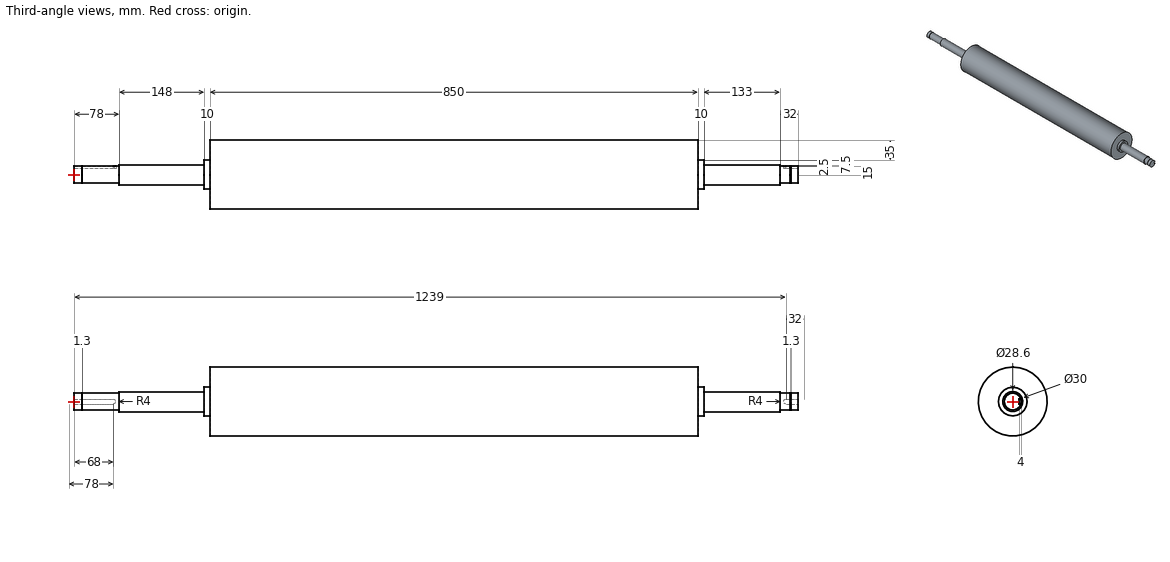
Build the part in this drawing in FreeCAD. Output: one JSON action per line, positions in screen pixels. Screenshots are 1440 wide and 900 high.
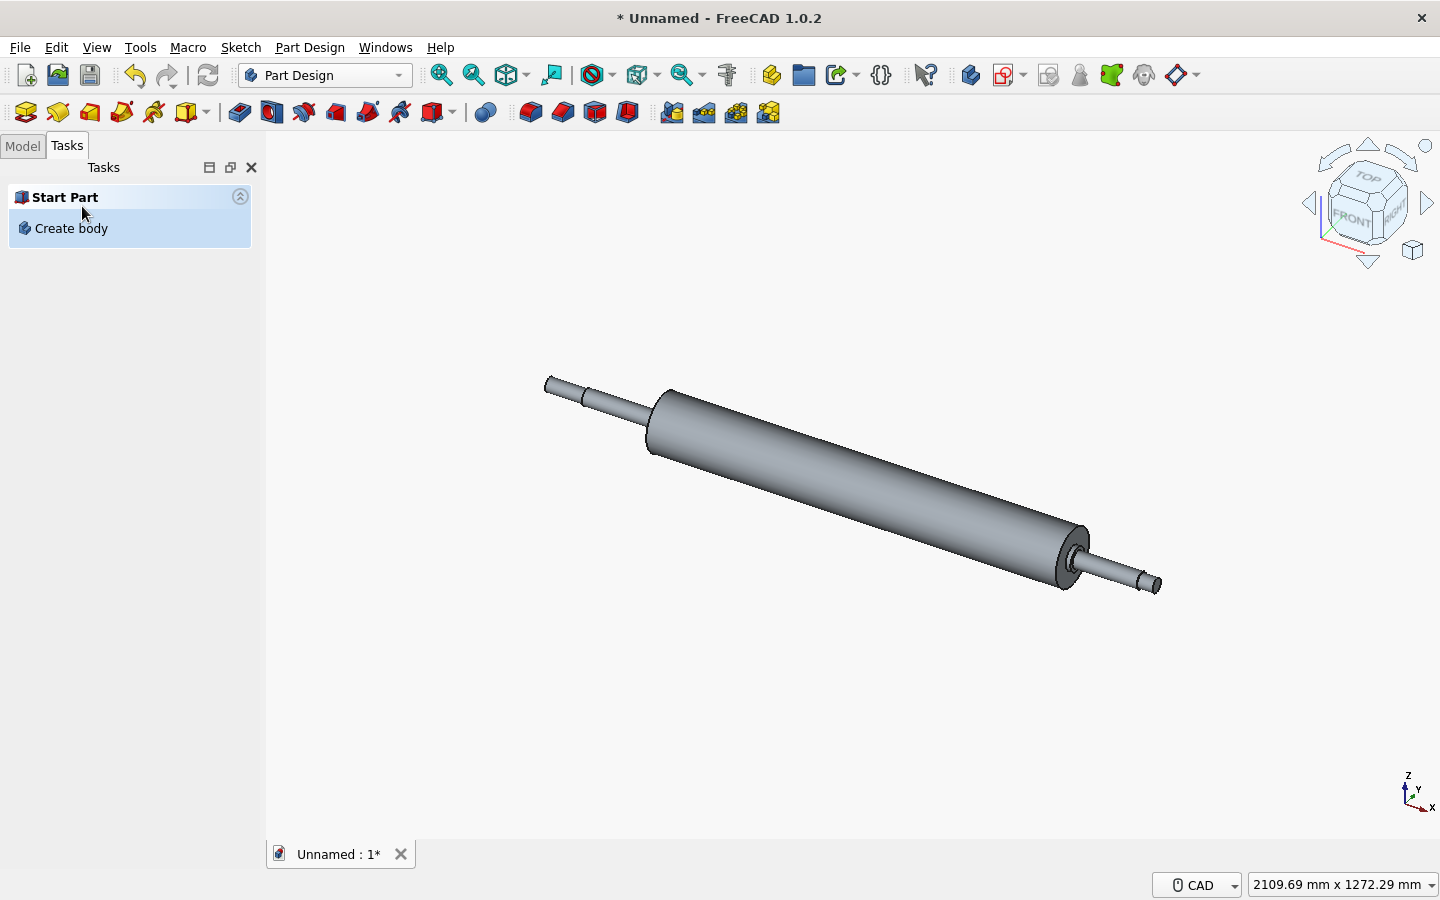
{"action": "left_click", "coordinate": [23, 145]}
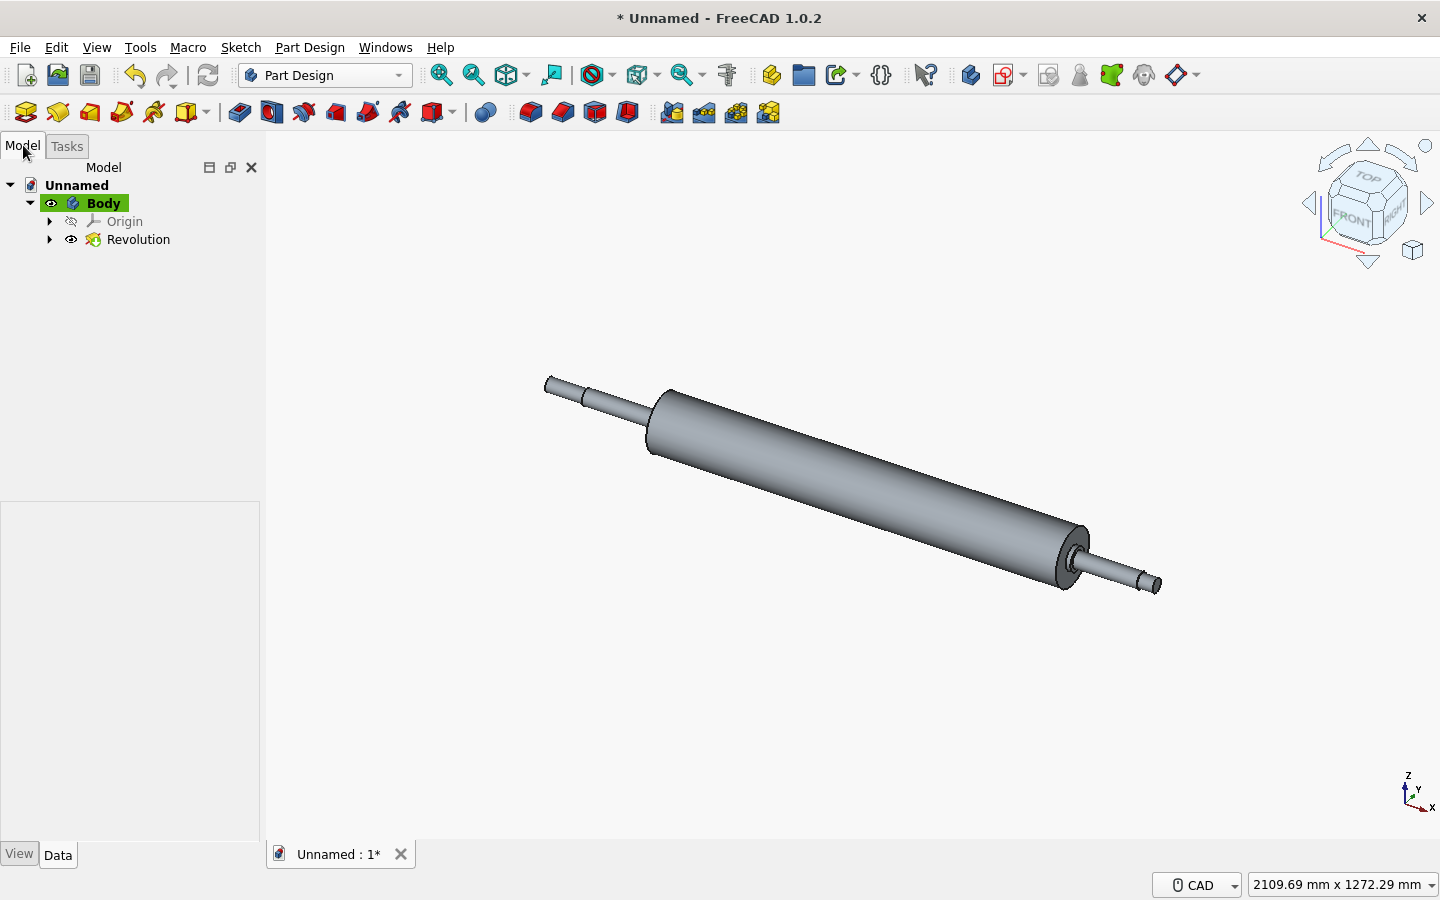
{"action": "left_click", "coordinate": [50, 221]}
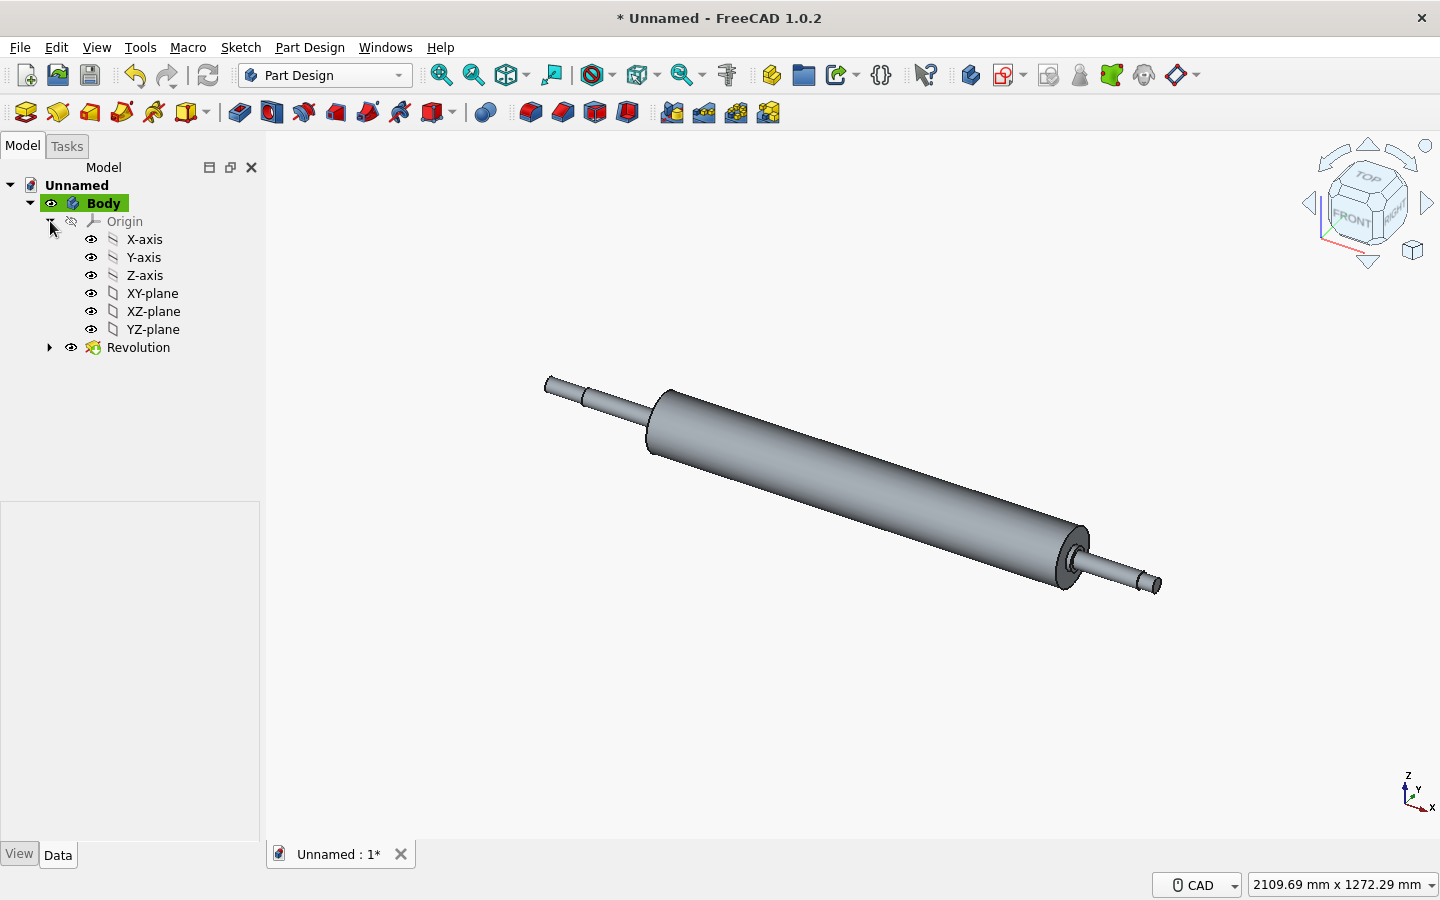
{"action": "left_click", "coordinate": [136, 311]}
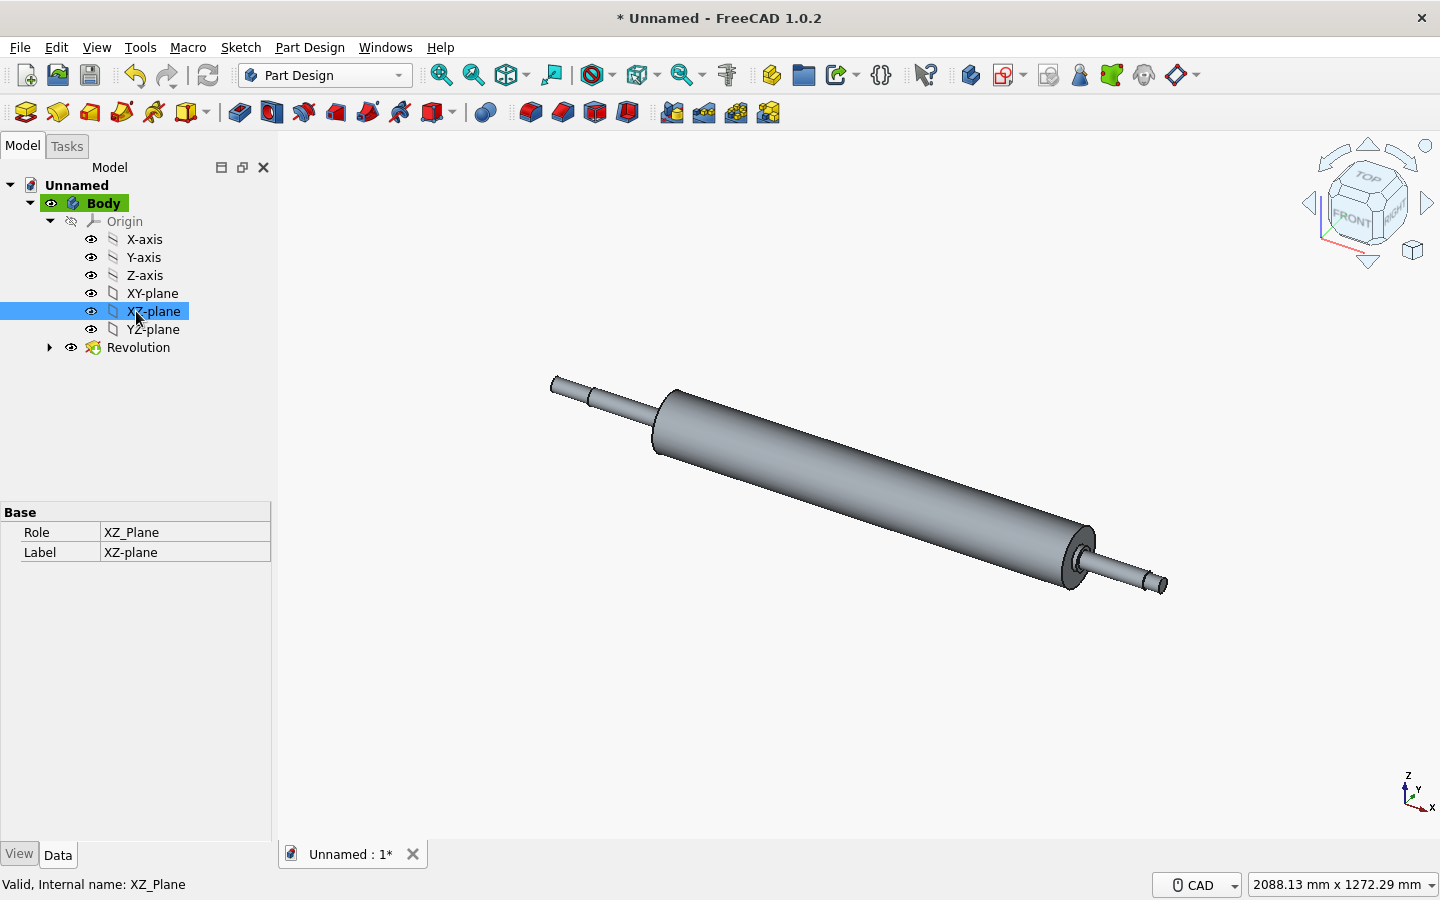
{"action": "left_click", "coordinate": [1176, 76]}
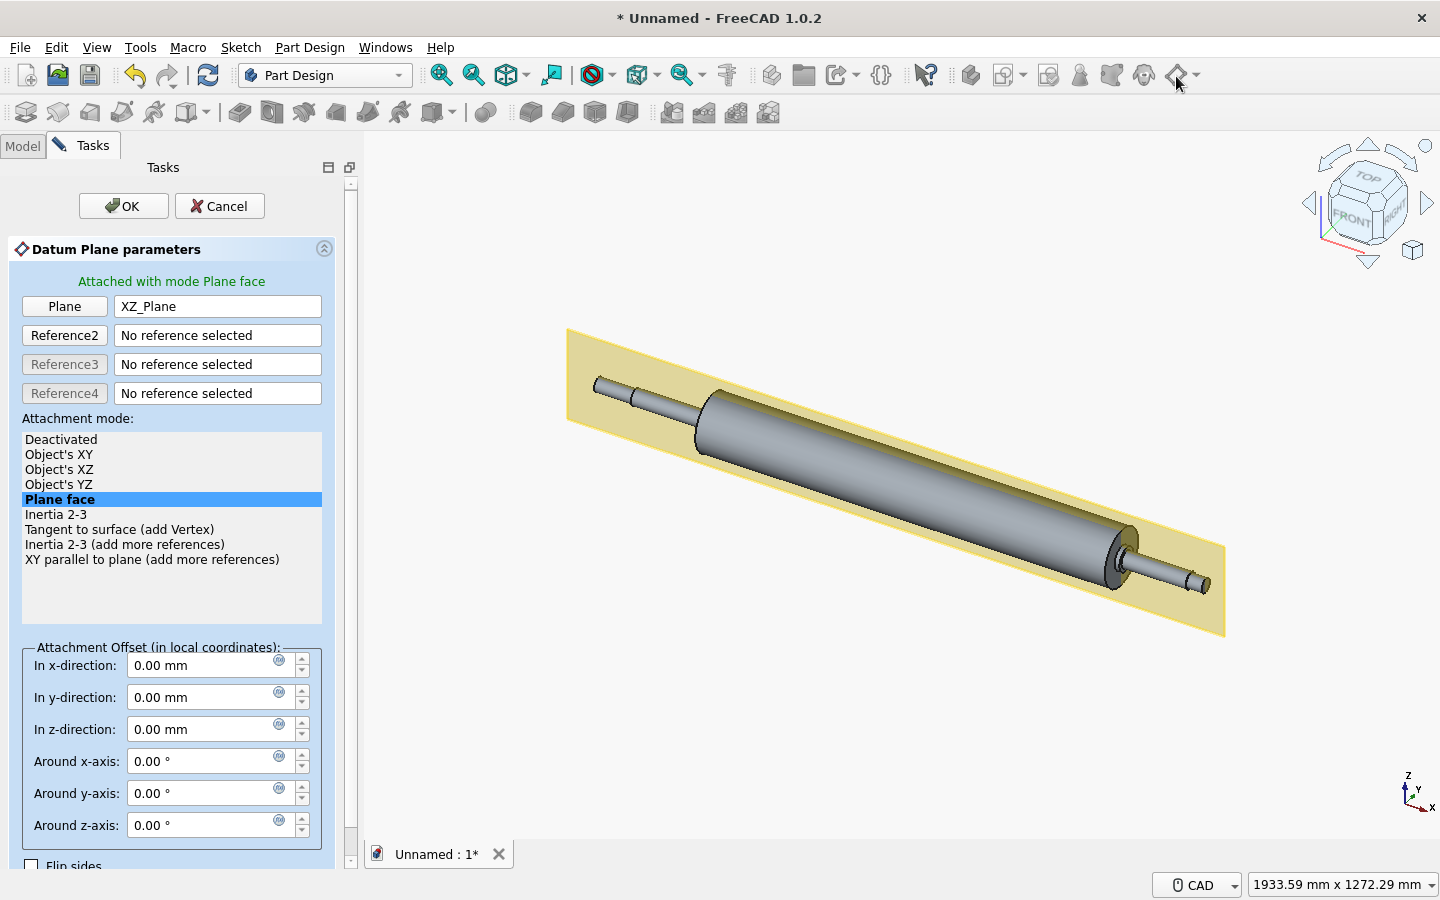
{"action": "triple_click", "coordinate": [210, 729]}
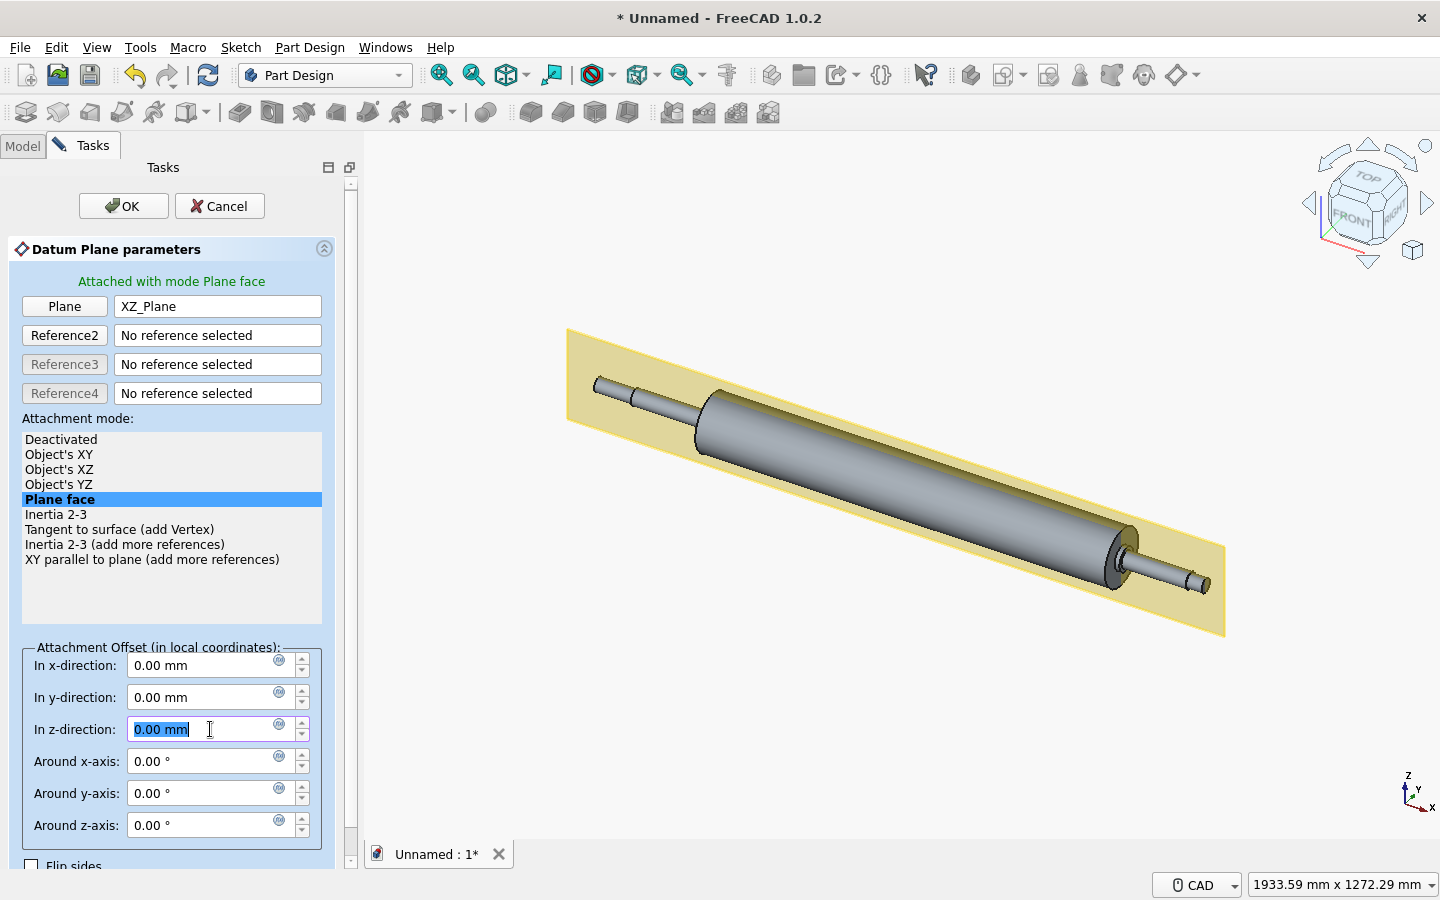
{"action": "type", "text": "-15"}
{"action": "key", "text": "Tab"}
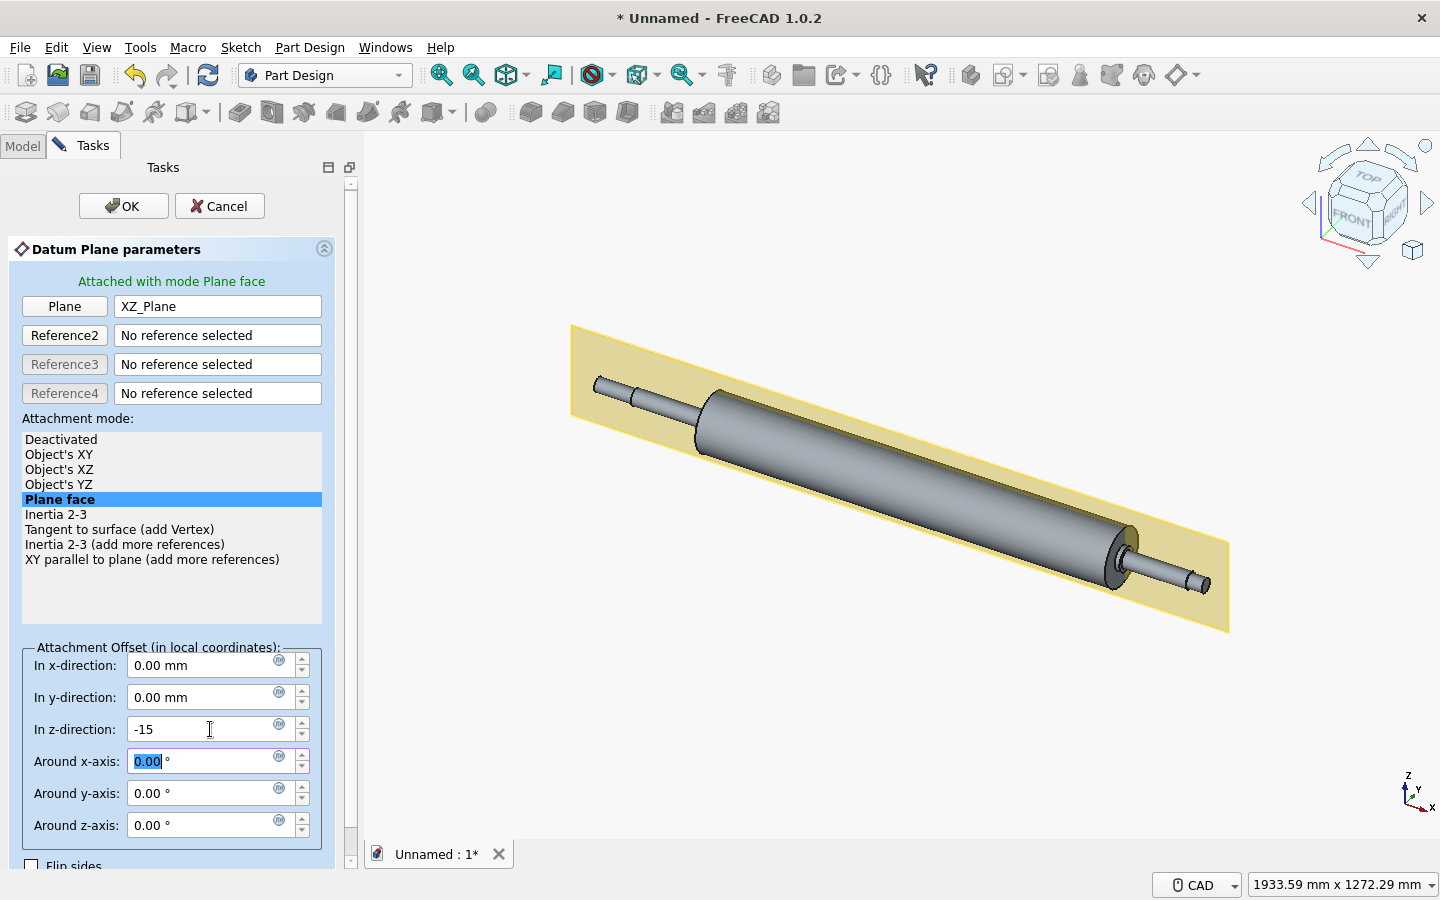
{"action": "left_click", "coordinate": [124, 206]}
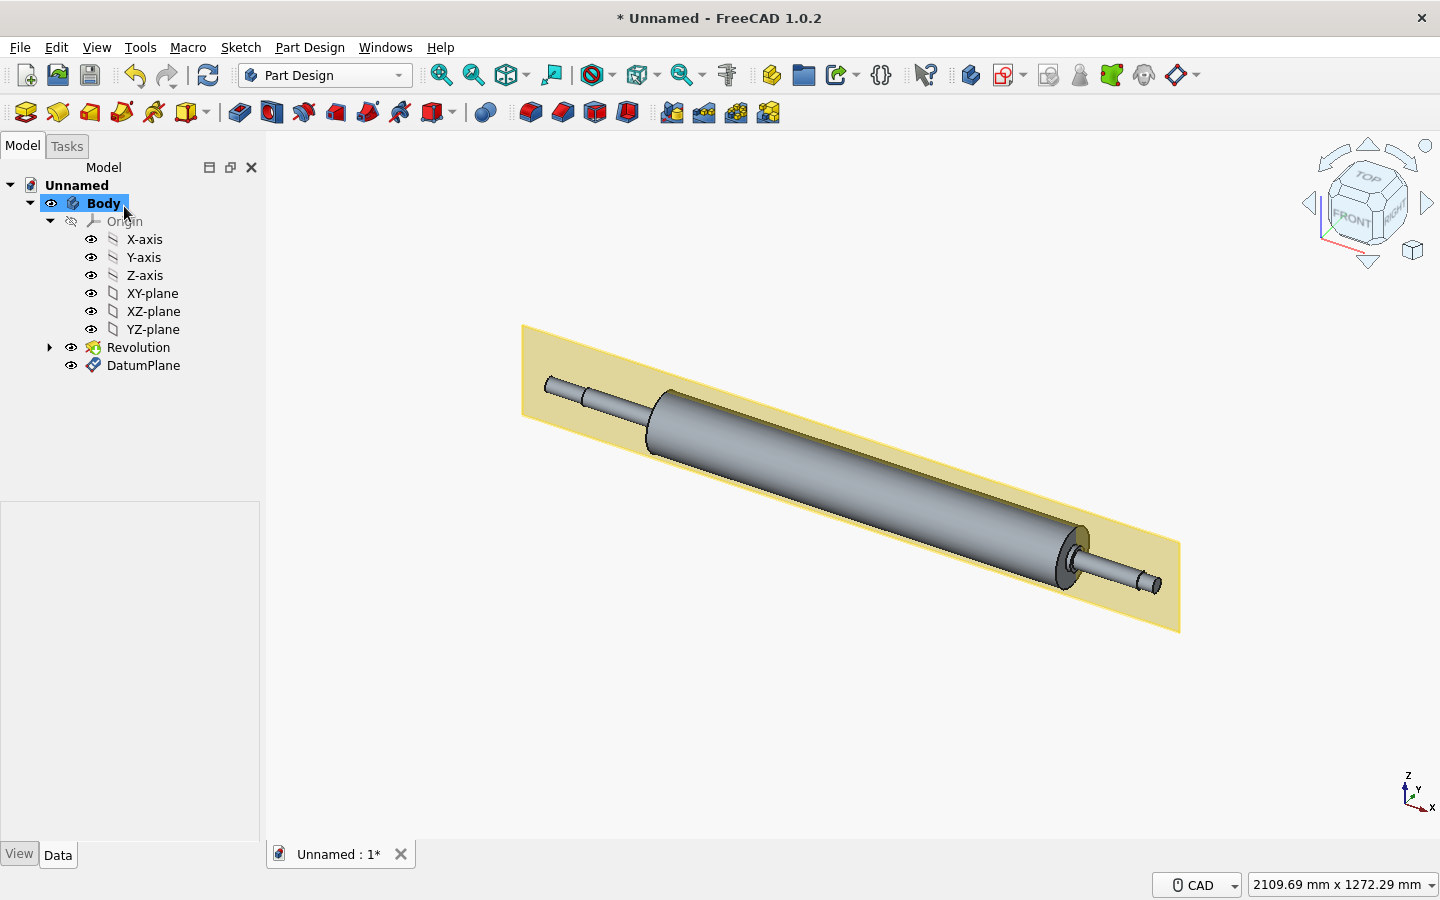
{"action": "left_click", "coordinate": [116, 365]}